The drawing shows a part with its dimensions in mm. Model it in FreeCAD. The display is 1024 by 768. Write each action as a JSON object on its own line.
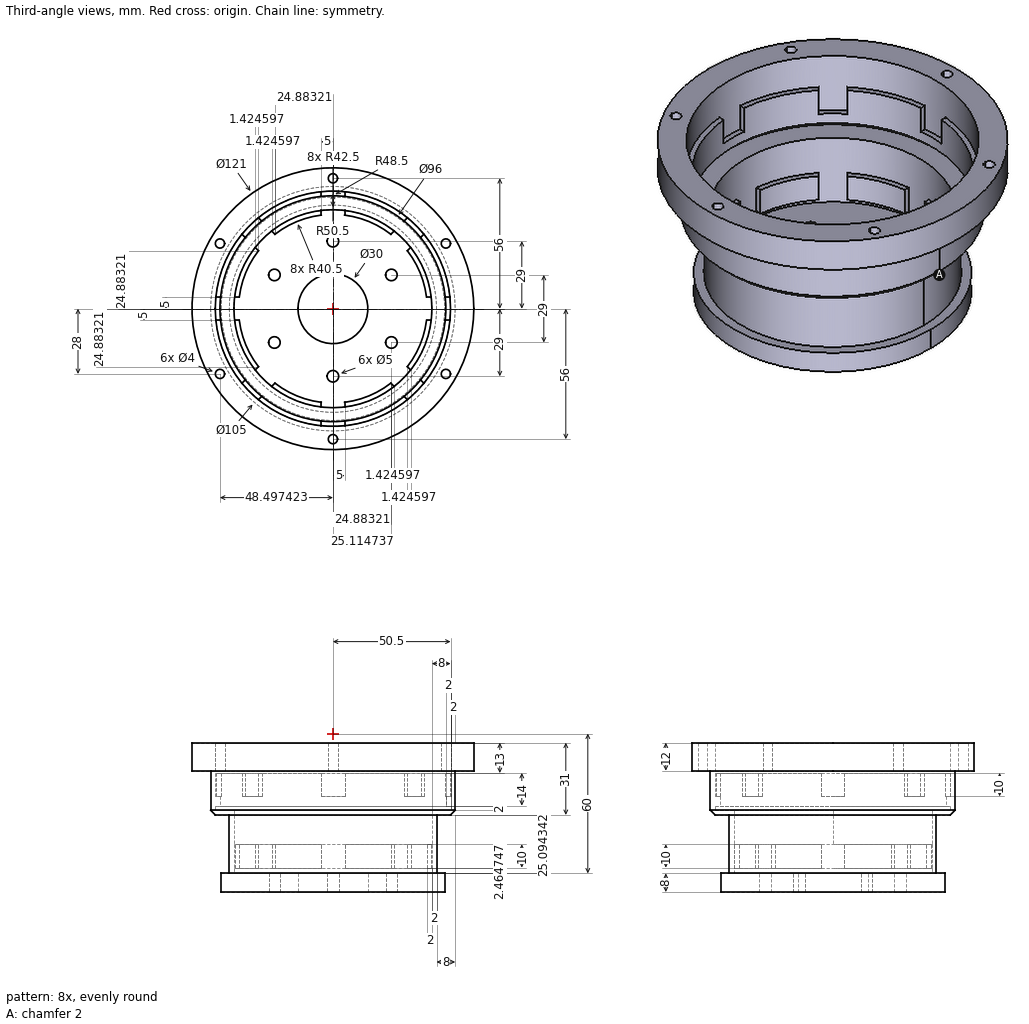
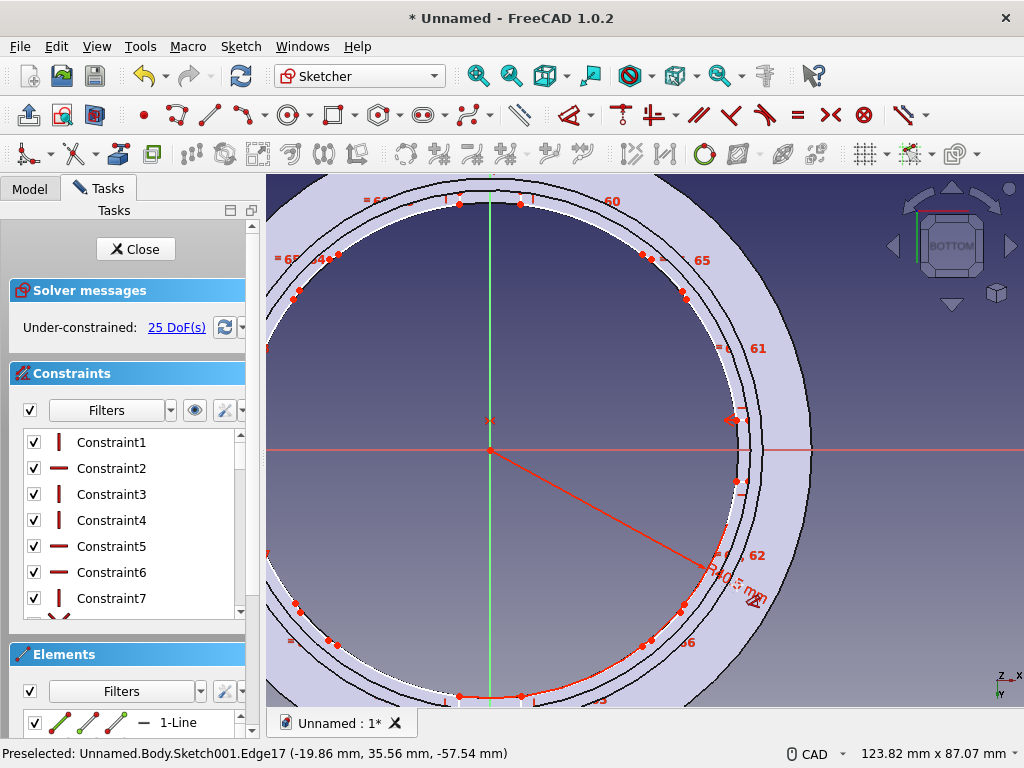
{"action": "left_click", "coordinate": [309, 621]}
{"action": "left_click", "coordinate": [298, 246]}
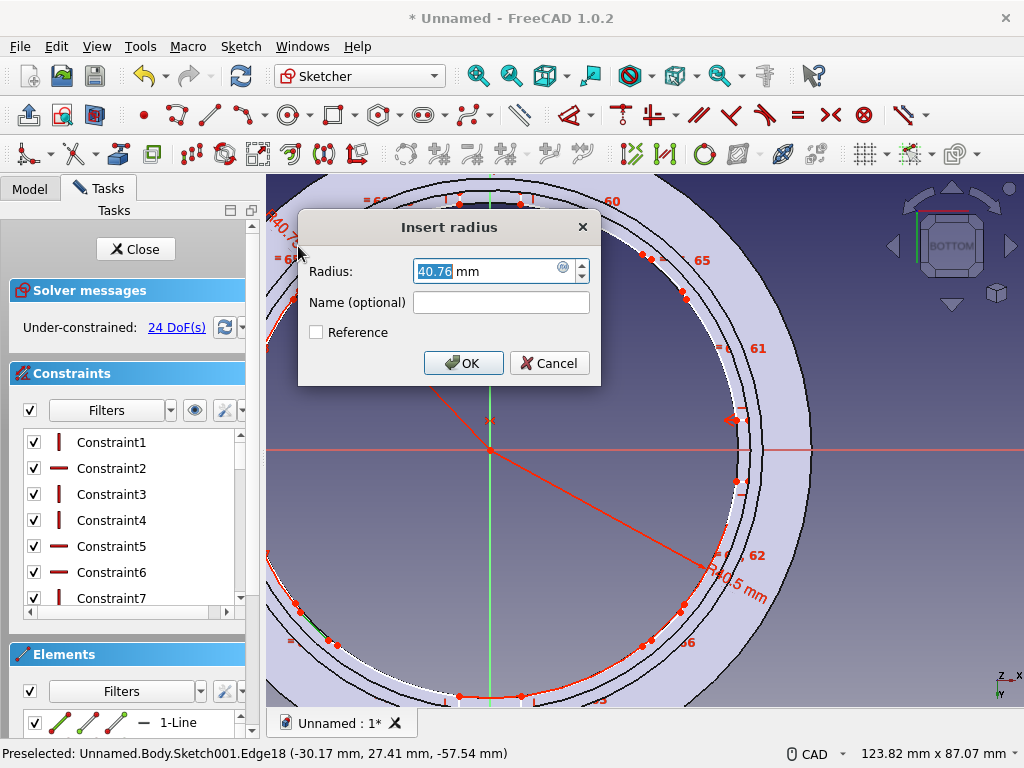
{"action": "type", "text": "42.5"}
{"action": "key", "text": "Return"}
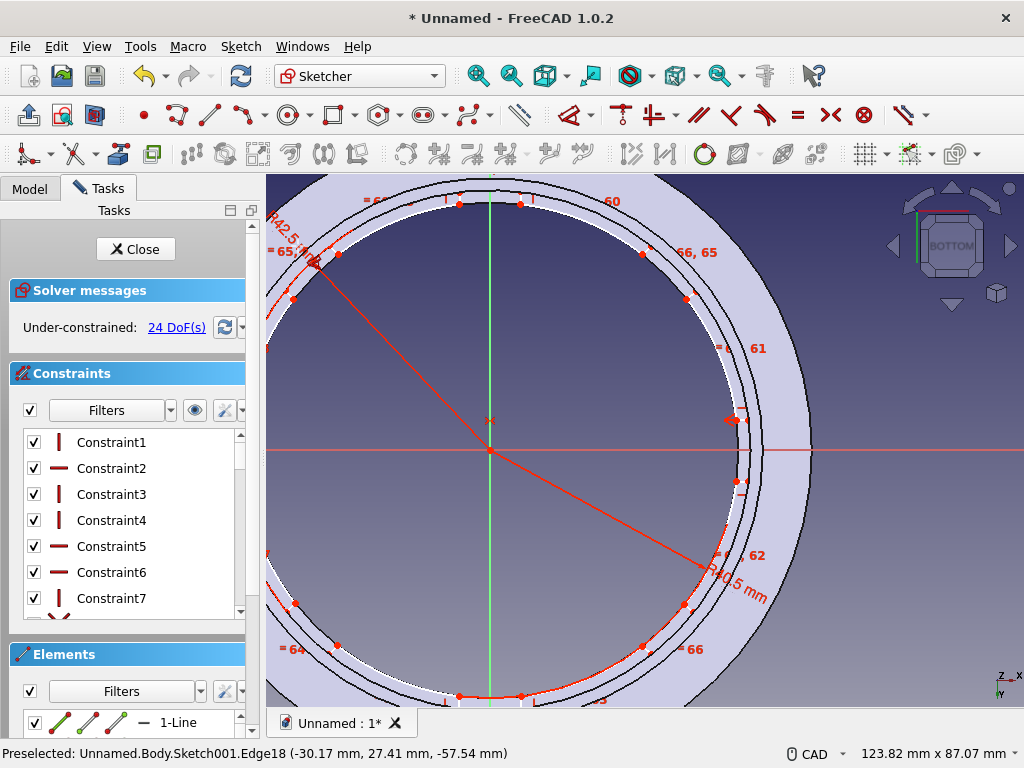
{"action": "scroll", "coordinate": [751, 420], "scroll_direction": "down", "scroll_amount": 2}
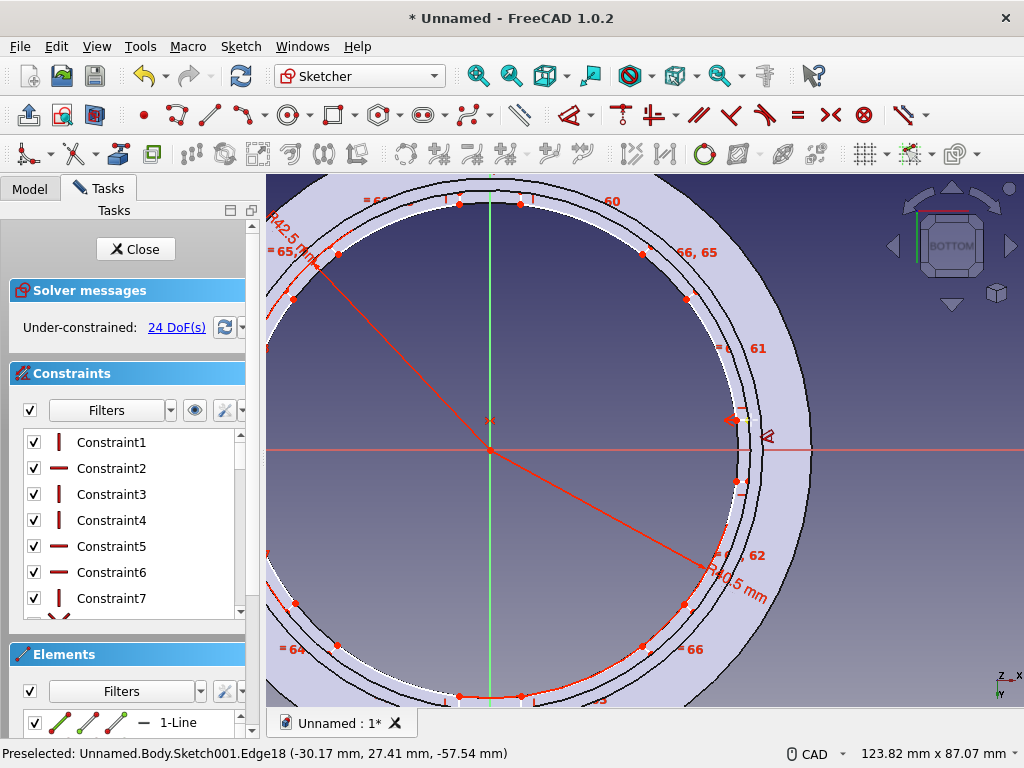
{"action": "scroll", "coordinate": [402, 433], "scroll_direction": "up", "scroll_amount": 3}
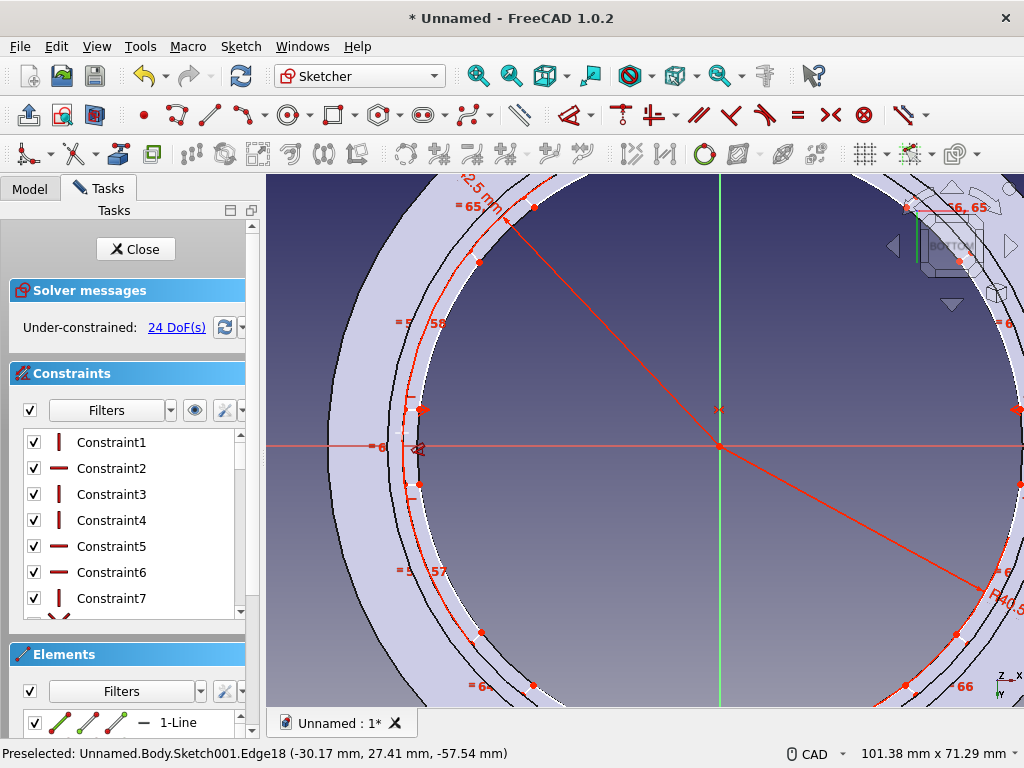
{"action": "left_click", "coordinate": [402, 432]}
{"action": "left_click", "coordinate": [370, 431]}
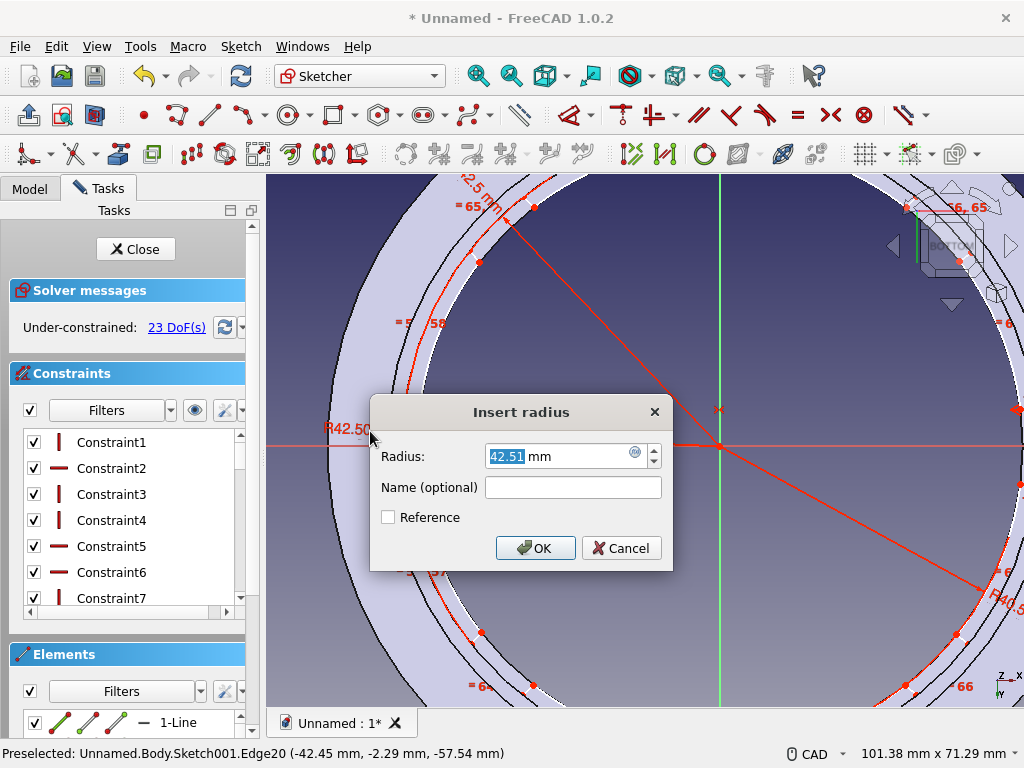
{"action": "type", "text": "42.5"}
{"action": "key", "text": "Return"}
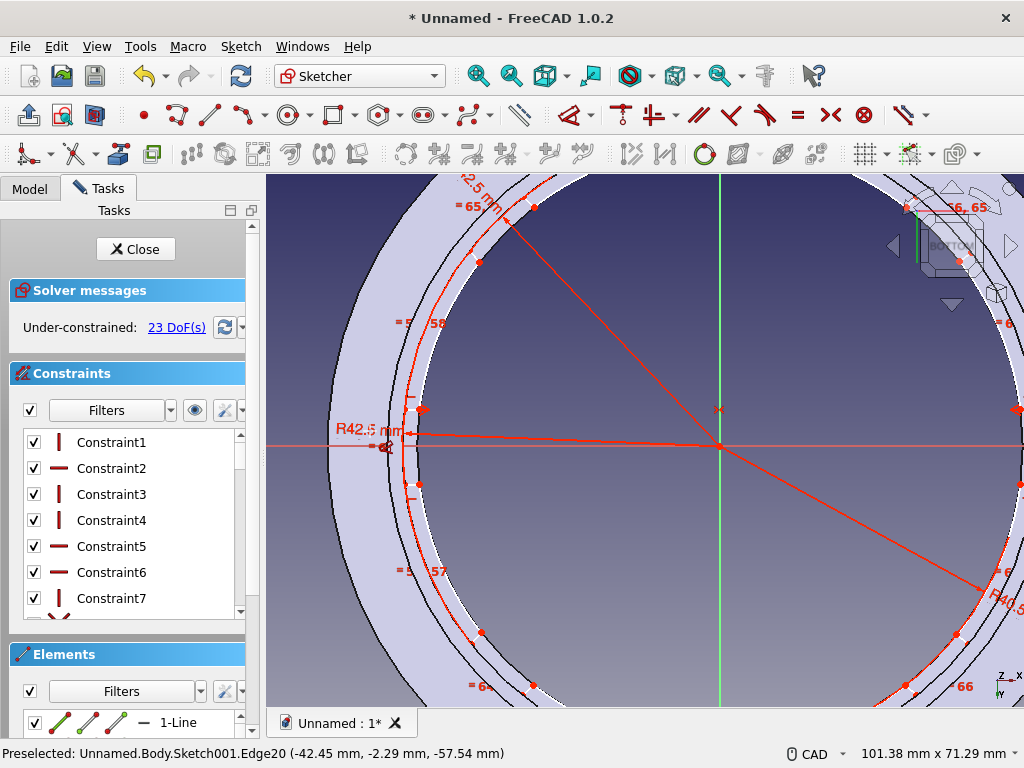
{"action": "scroll", "coordinate": [402, 433], "scroll_direction": "down", "scroll_amount": 3}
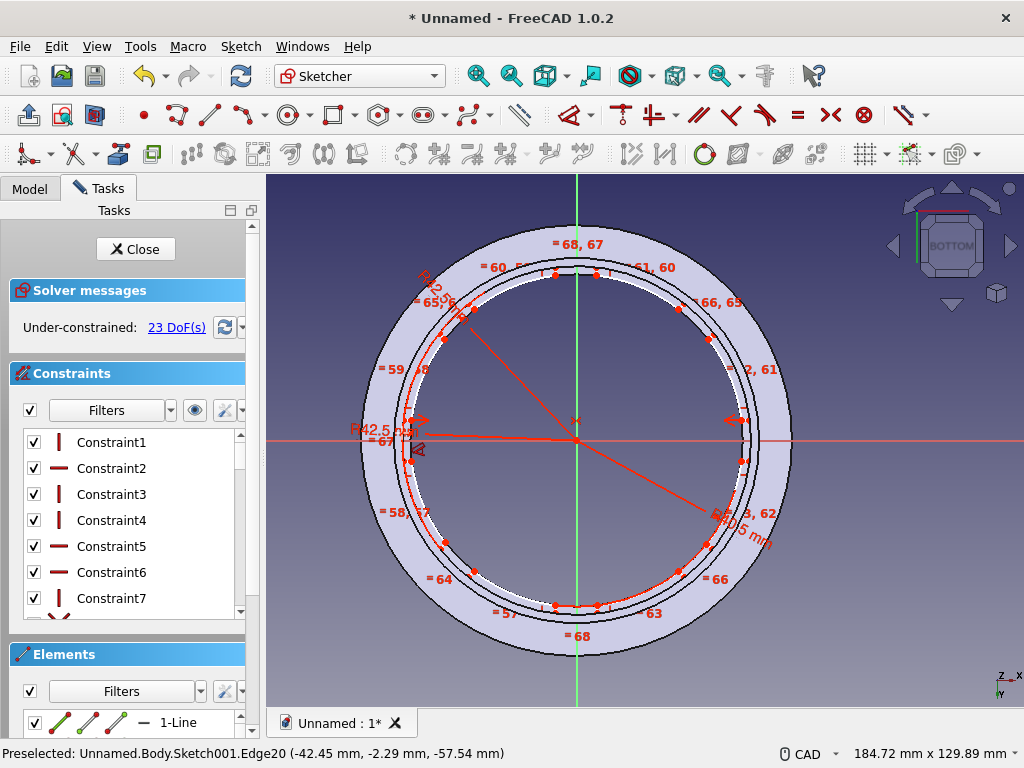
{"action": "scroll", "coordinate": [556, 614], "scroll_direction": "up", "scroll_amount": 4}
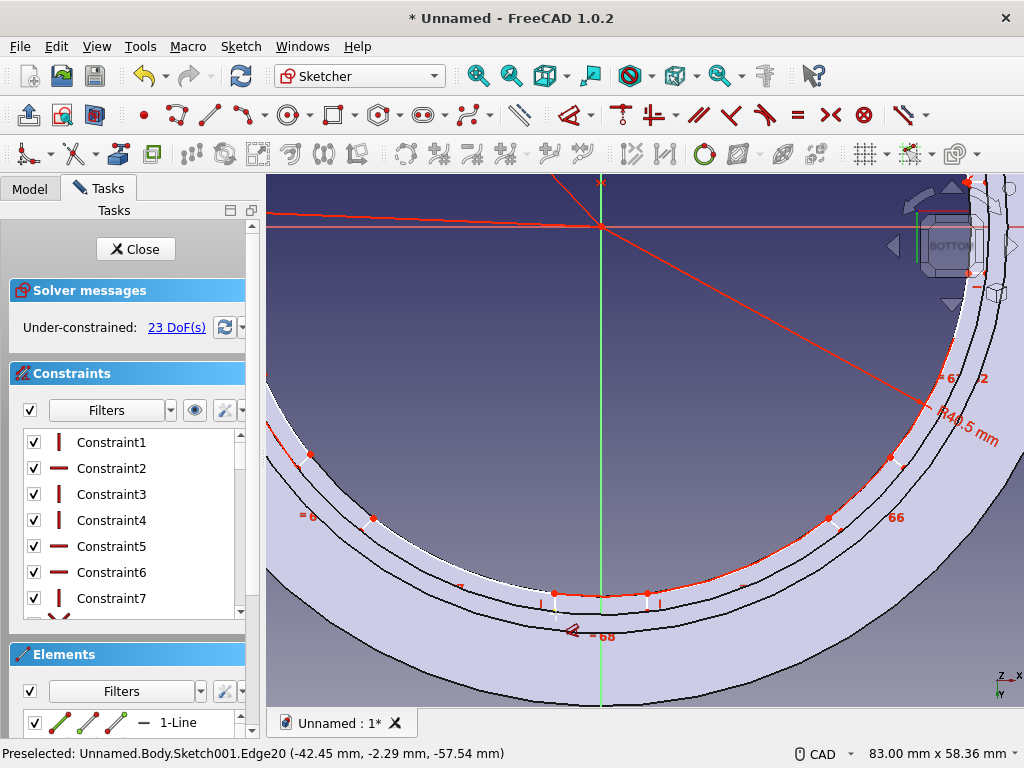
{"action": "left_click", "coordinate": [555, 612]}
{"action": "left_click", "coordinate": [578, 646]}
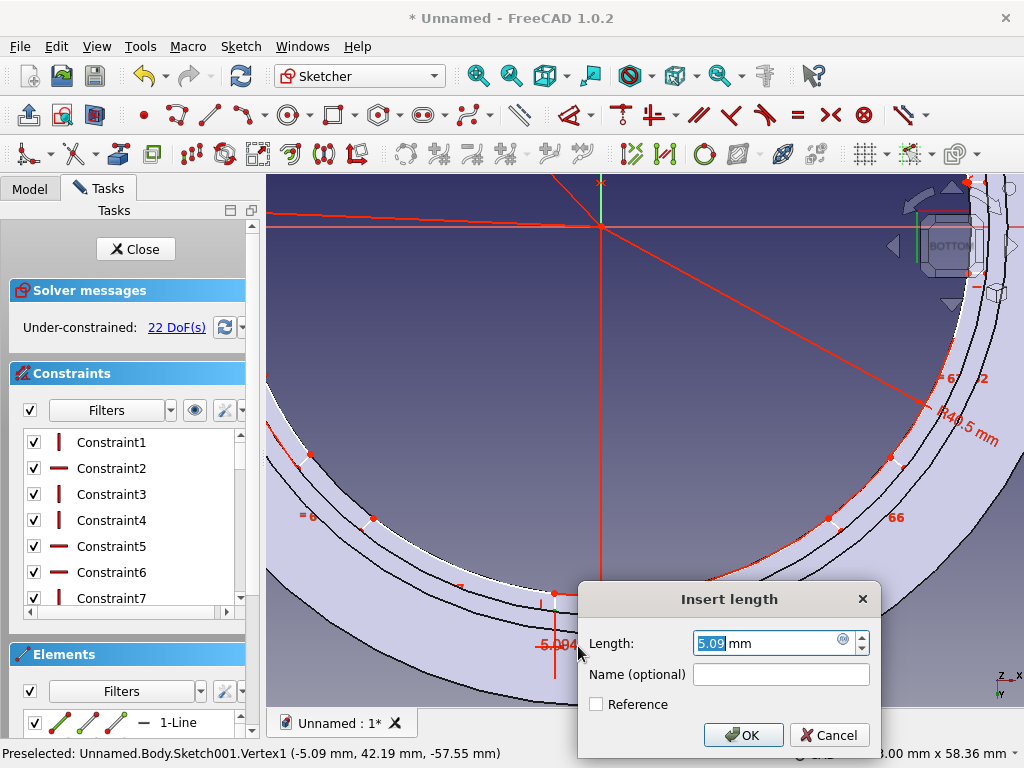
{"action": "type", "text": "5"}
{"action": "key", "text": "Return"}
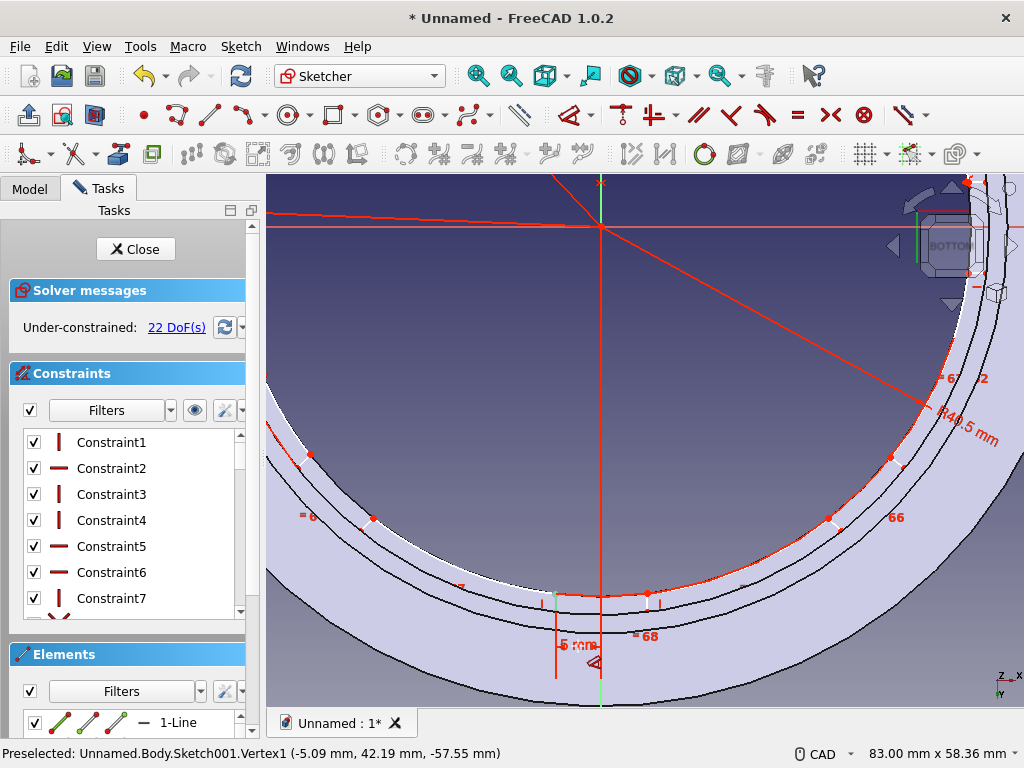
{"action": "scroll", "coordinate": [556, 615], "scroll_direction": "down", "scroll_amount": 4}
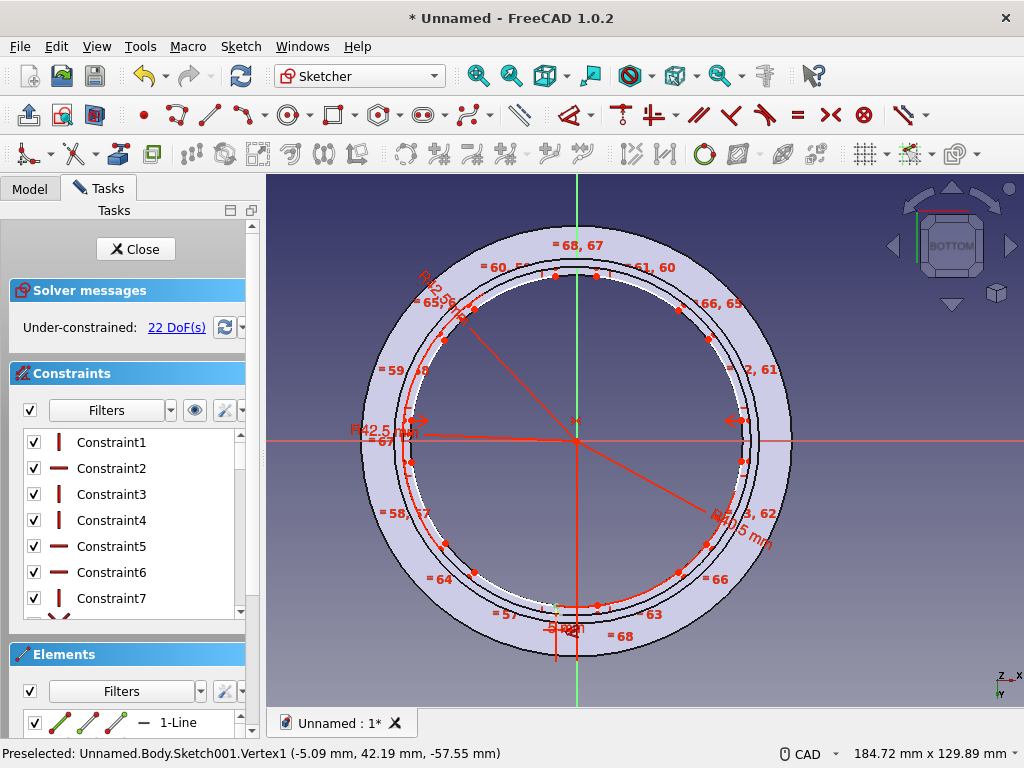
{"action": "scroll", "coordinate": [412, 462], "scroll_direction": "up", "scroll_amount": 4}